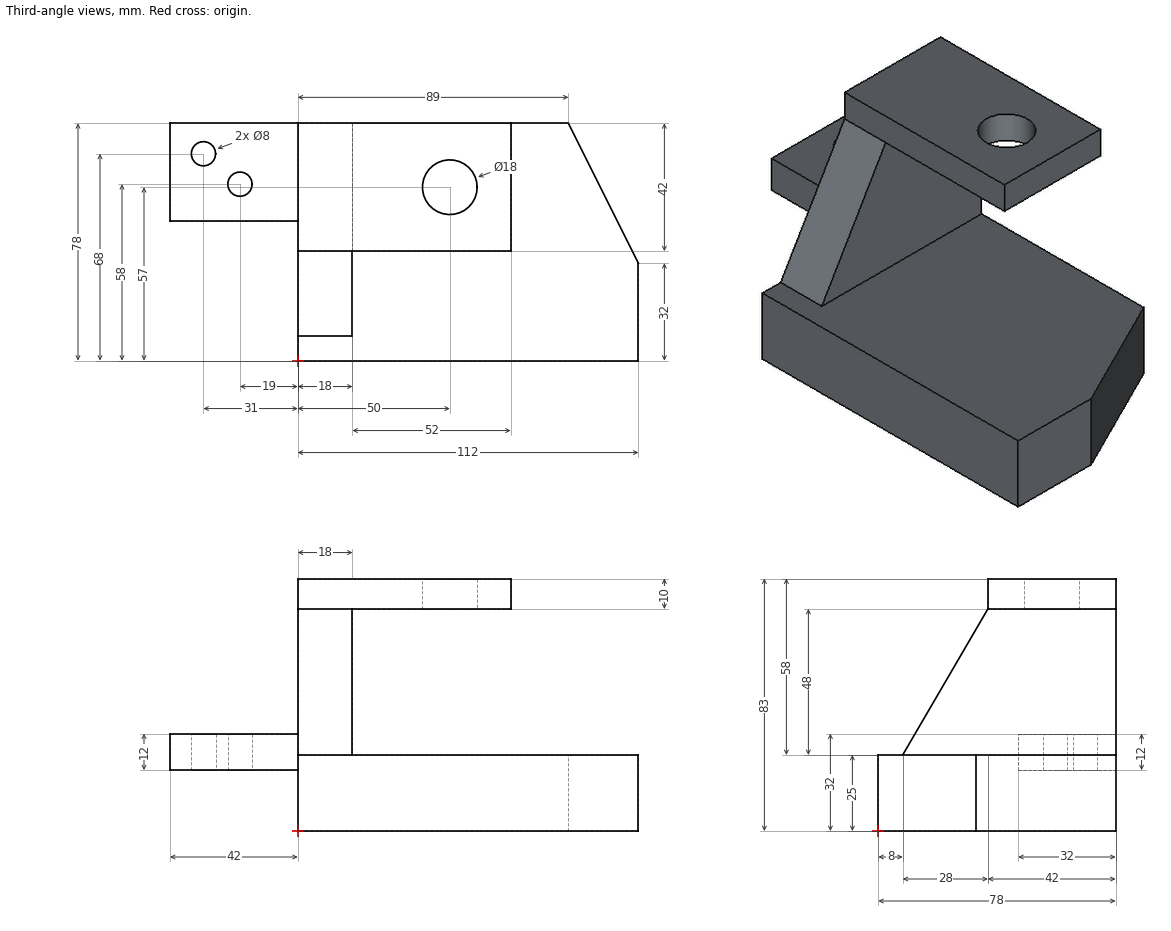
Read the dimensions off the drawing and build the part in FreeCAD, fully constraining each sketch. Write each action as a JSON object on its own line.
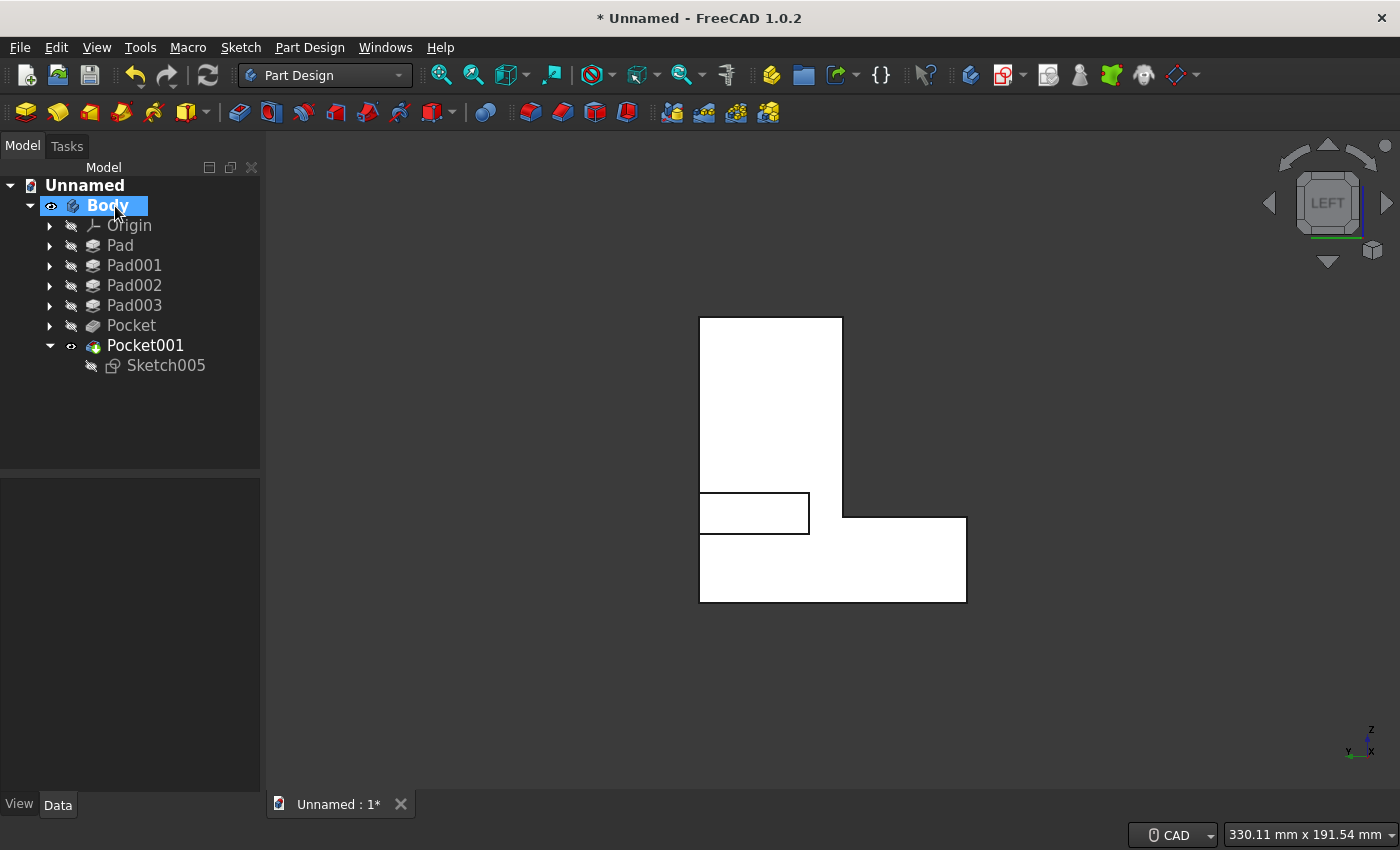
{"action": "key", "text": "v f"}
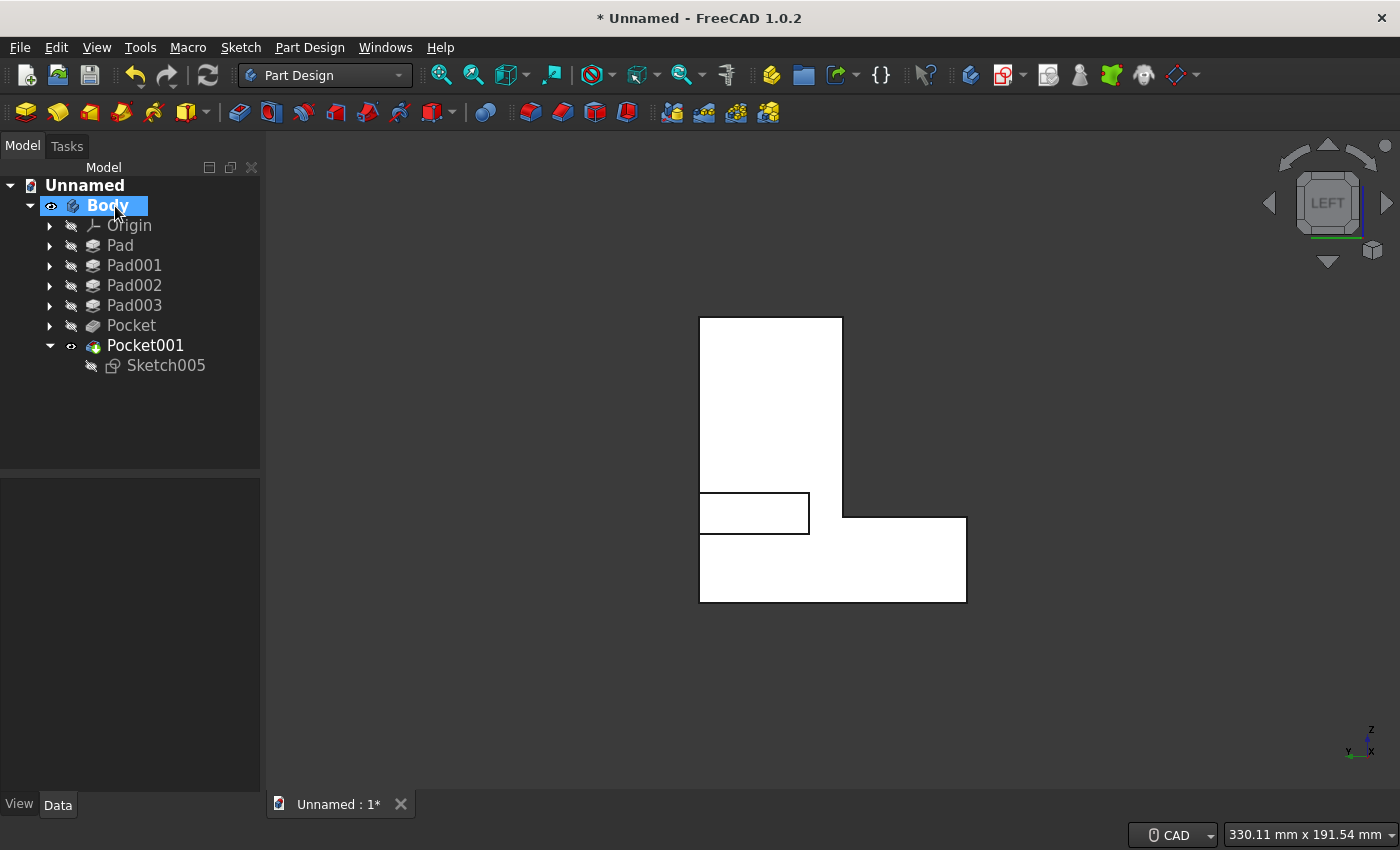
{"action": "left_click", "coordinate": [756, 378]}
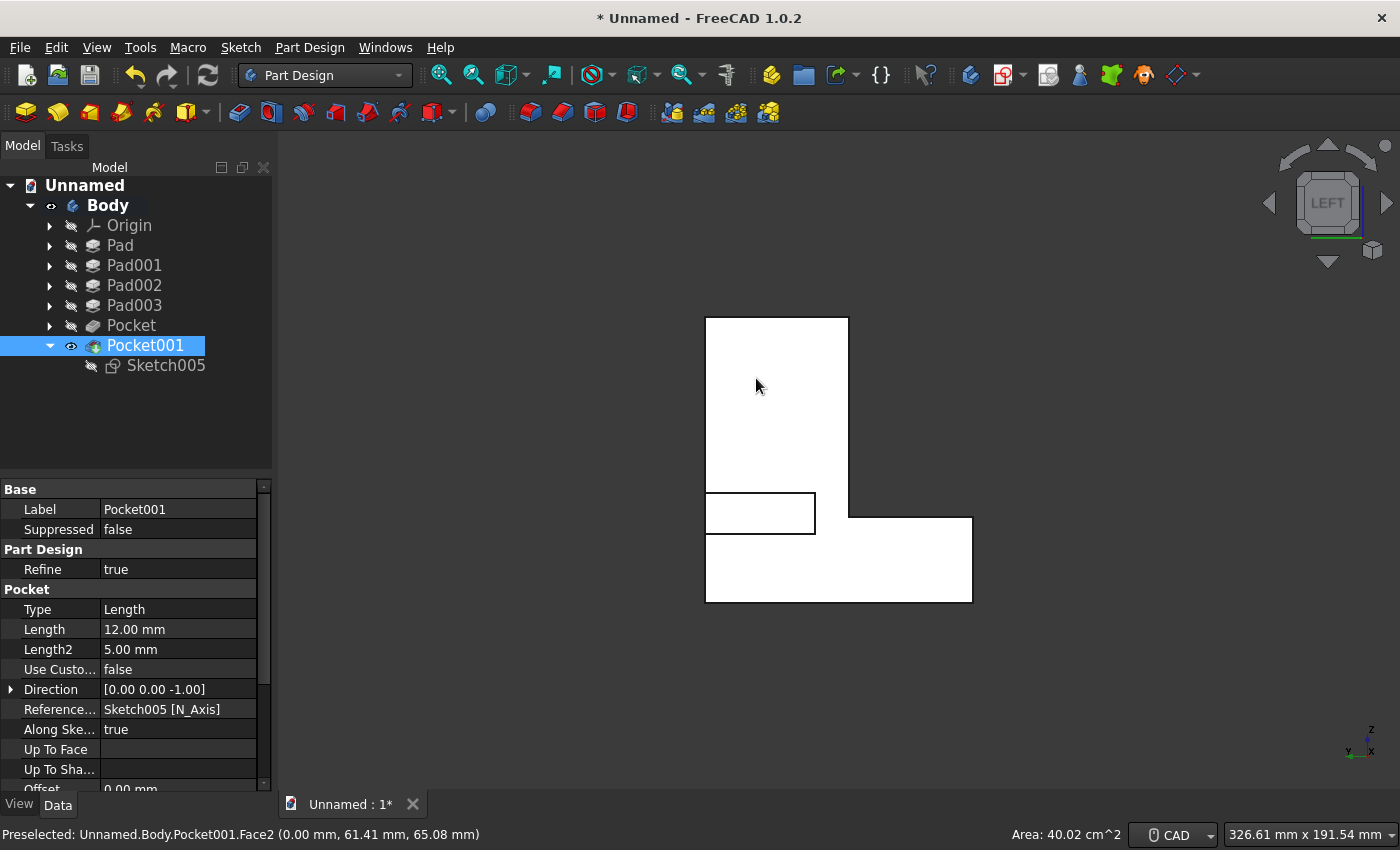
{"action": "left_click", "coordinate": [1004, 76]}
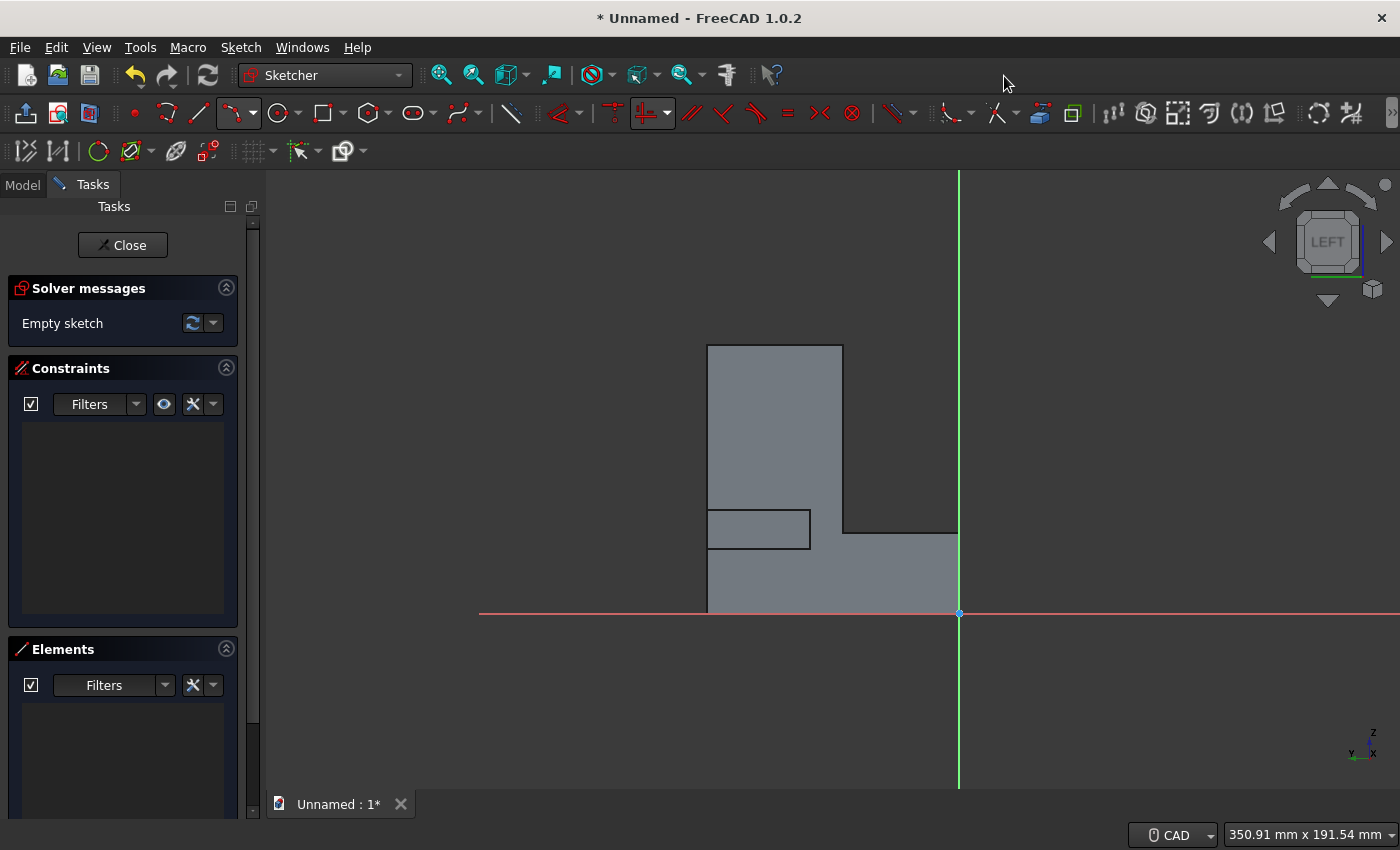
{"action": "key", "text": "q s"}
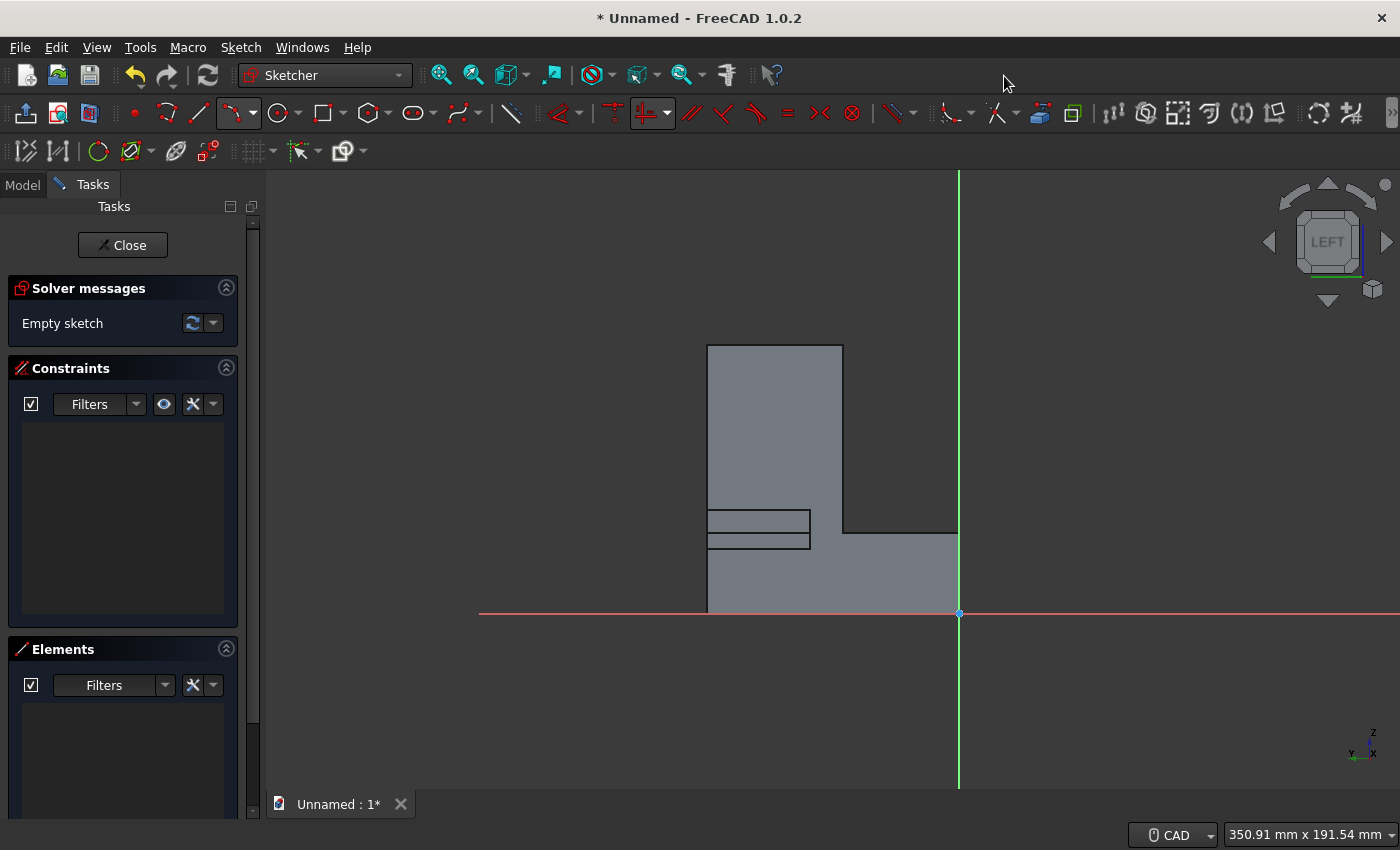
{"action": "scroll", "coordinate": [1067, 515], "scroll_direction": "up", "scroll_amount": 3}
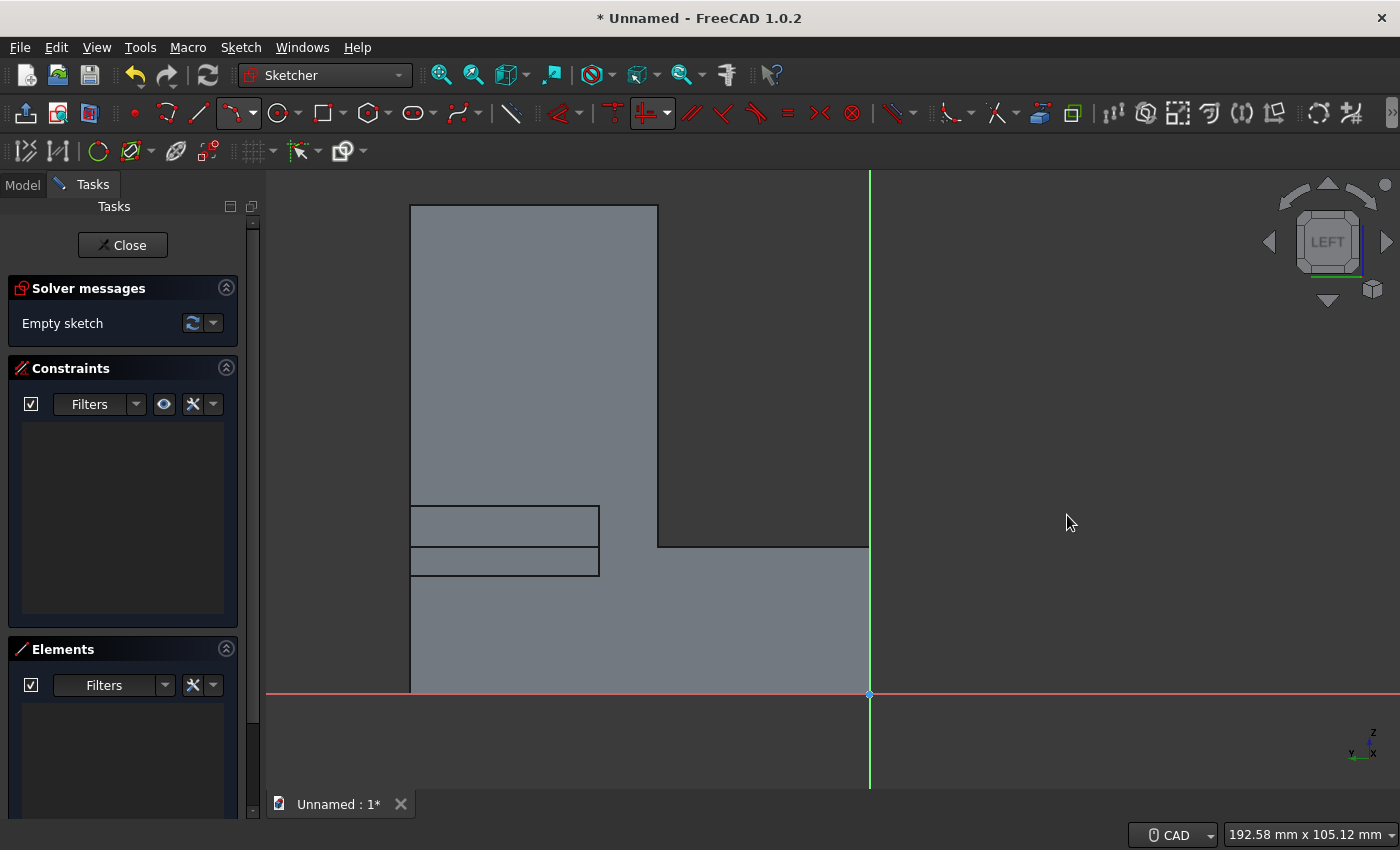
{"action": "key", "text": "g m"}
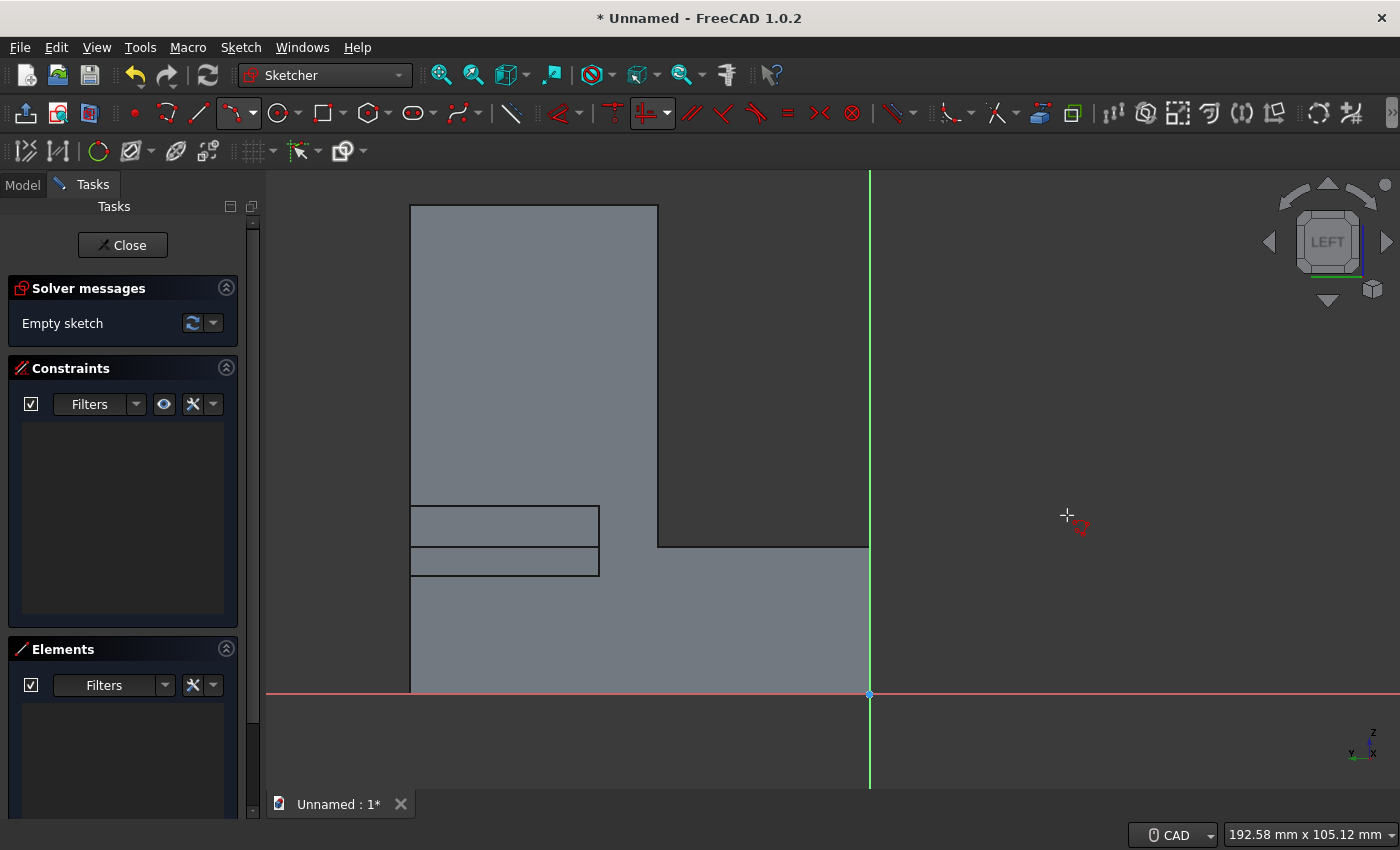
{"action": "left_click", "coordinate": [823, 547]}
{"action": "left_click", "coordinate": [658, 264]}
{"action": "left_click", "coordinate": [658, 547]}
{"action": "left_click", "coordinate": [823, 548]}
{"action": "key", "text": "Escape"}
{"action": "key", "text": "Escape"}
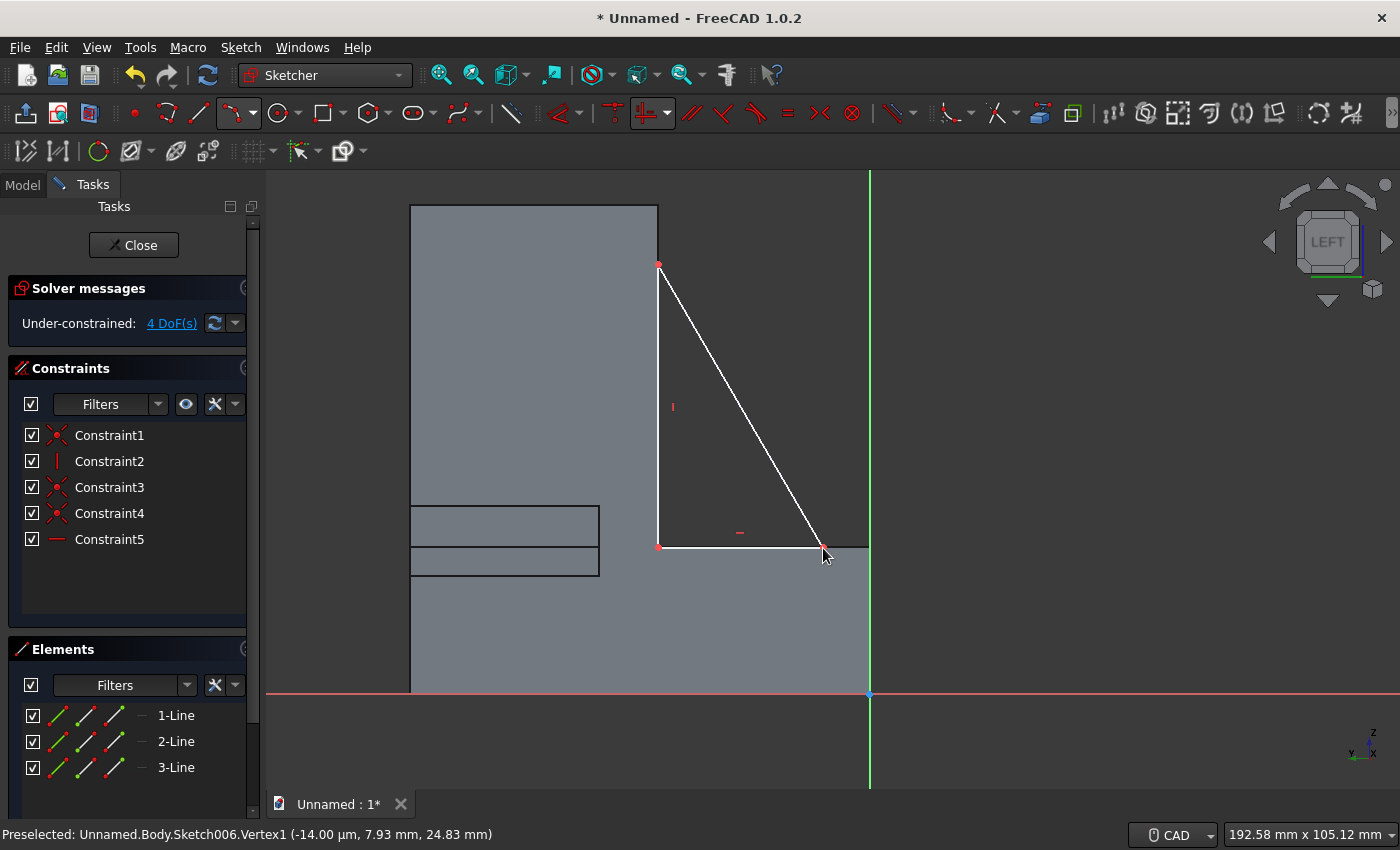
{"action": "key", "text": "d"}